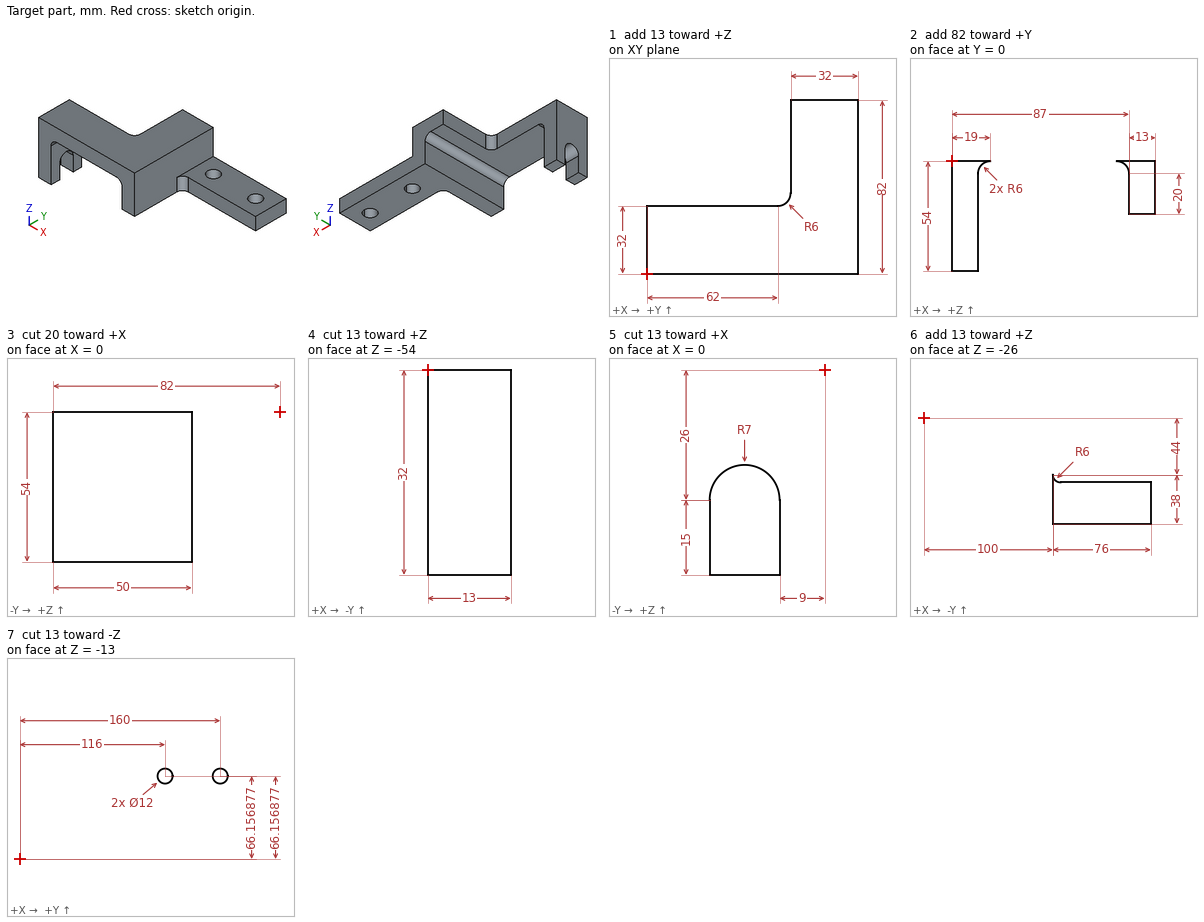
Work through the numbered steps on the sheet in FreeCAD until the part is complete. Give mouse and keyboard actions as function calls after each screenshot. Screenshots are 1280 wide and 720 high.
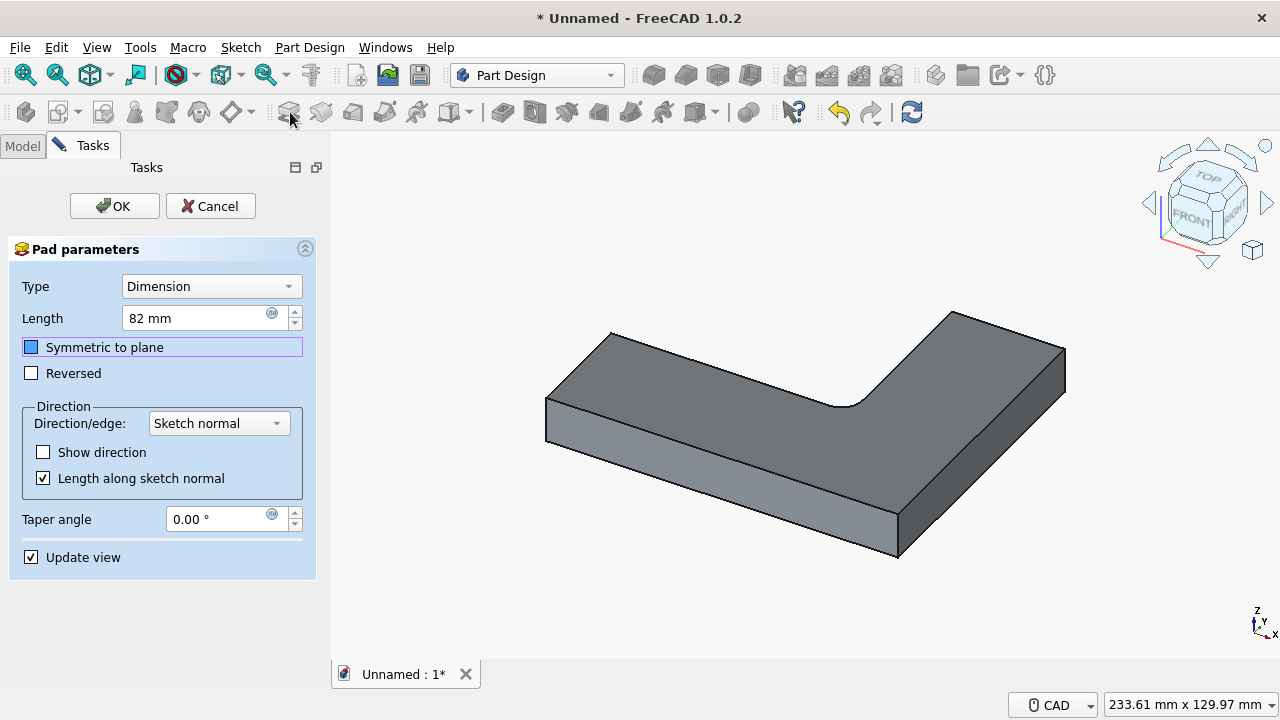
click(30, 373)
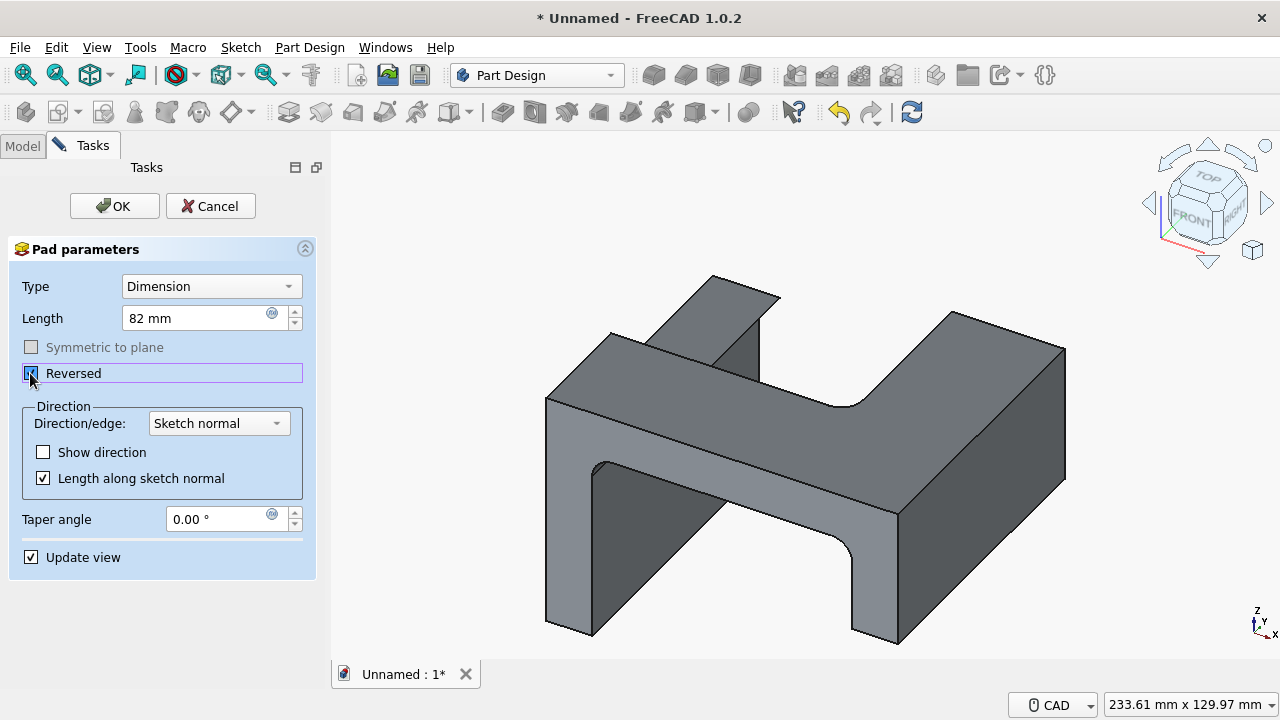
click(115, 206)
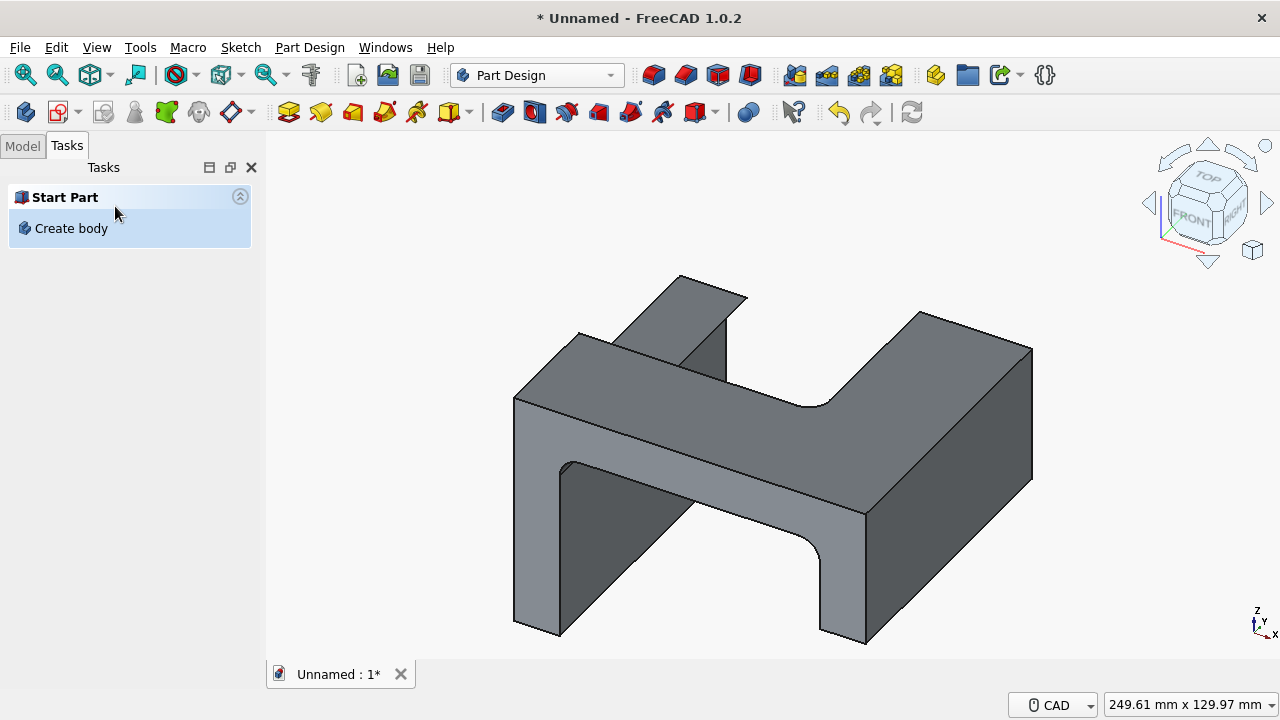
click(26, 76)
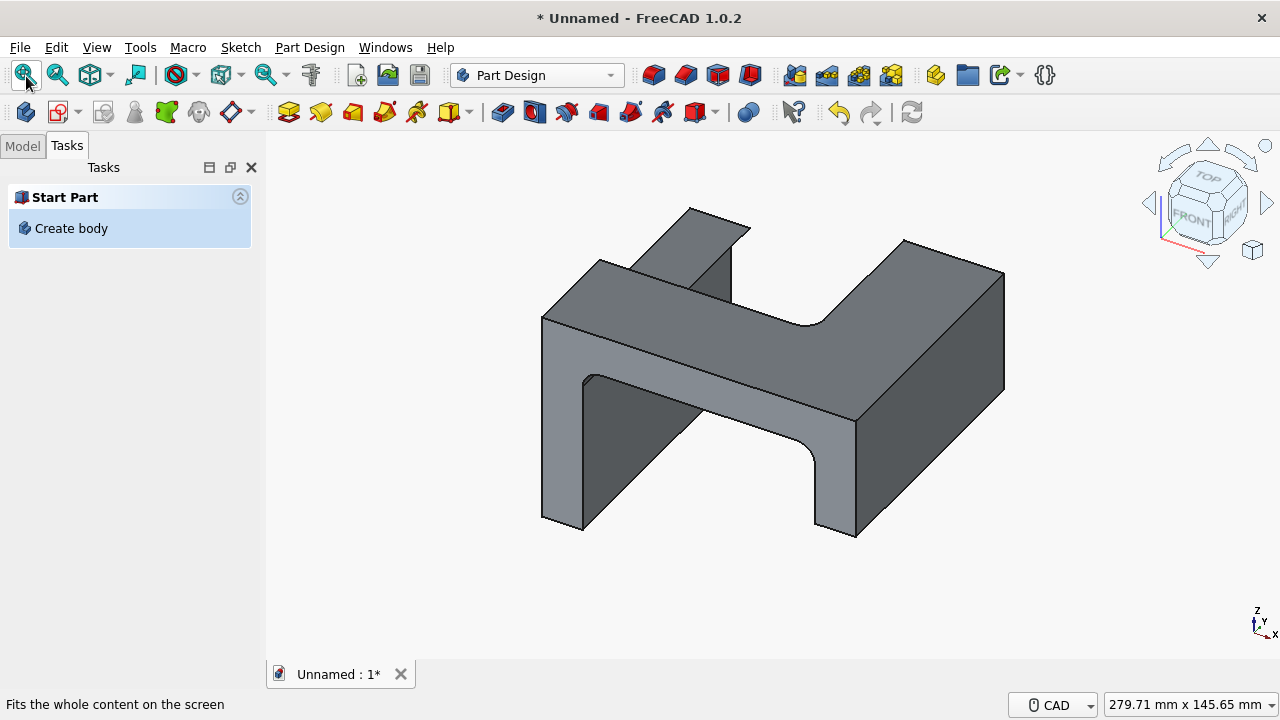
key(6)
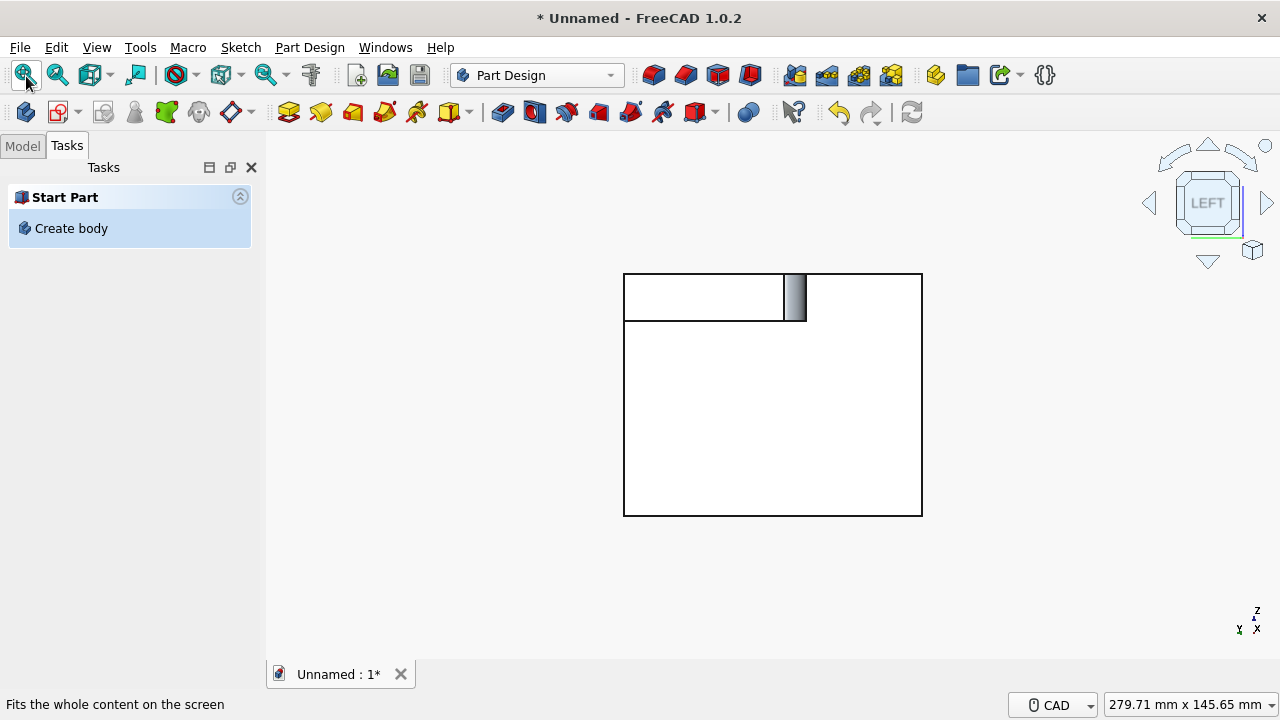
click(731, 429)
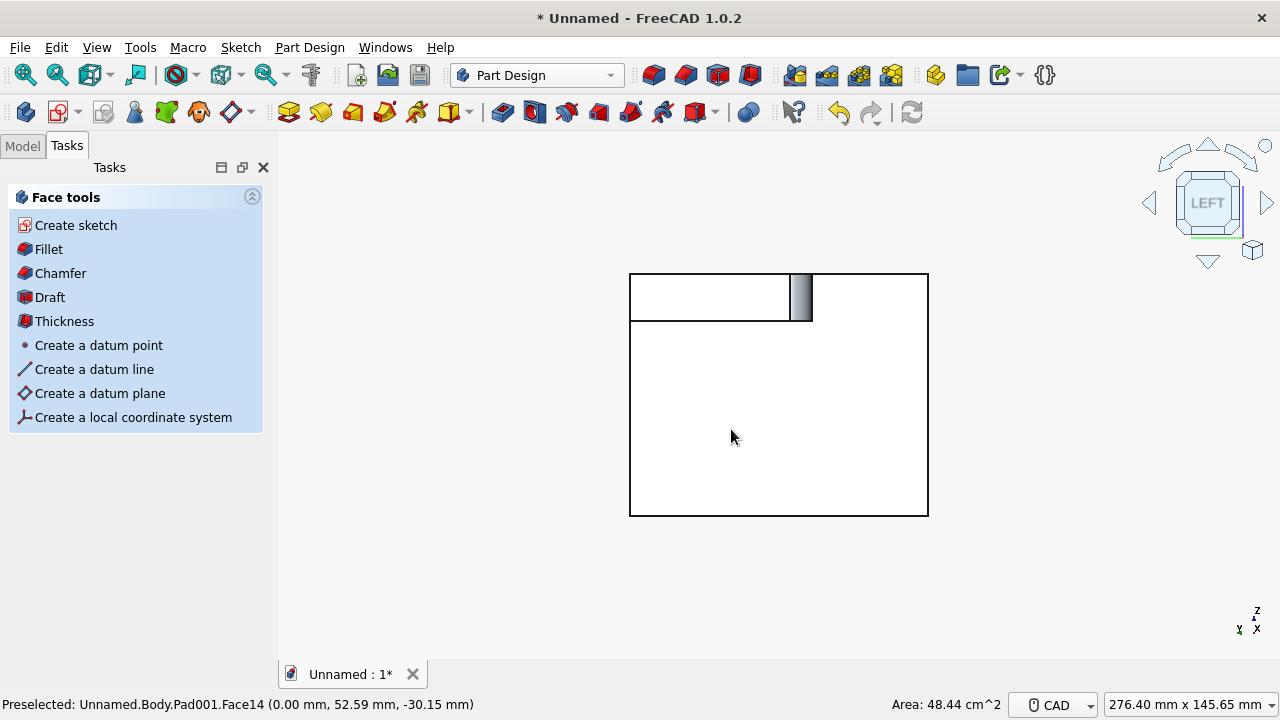
click(58, 112)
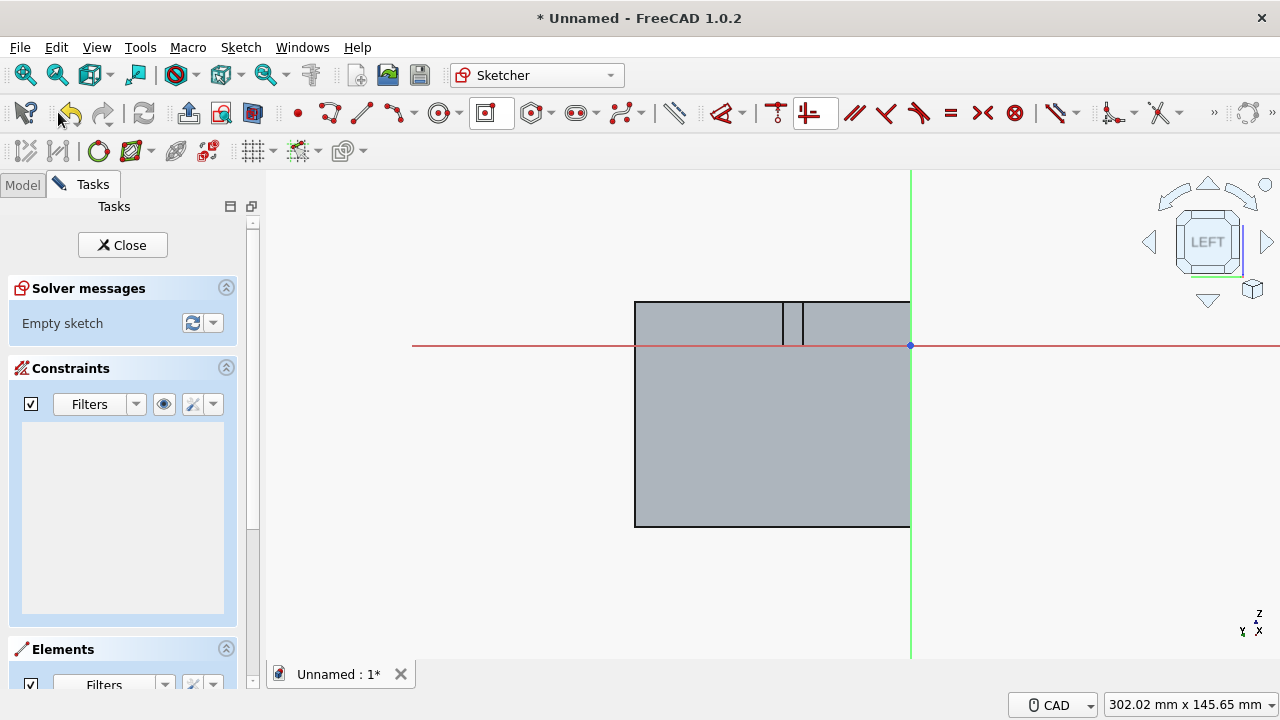
scroll(856, 463, up, 3)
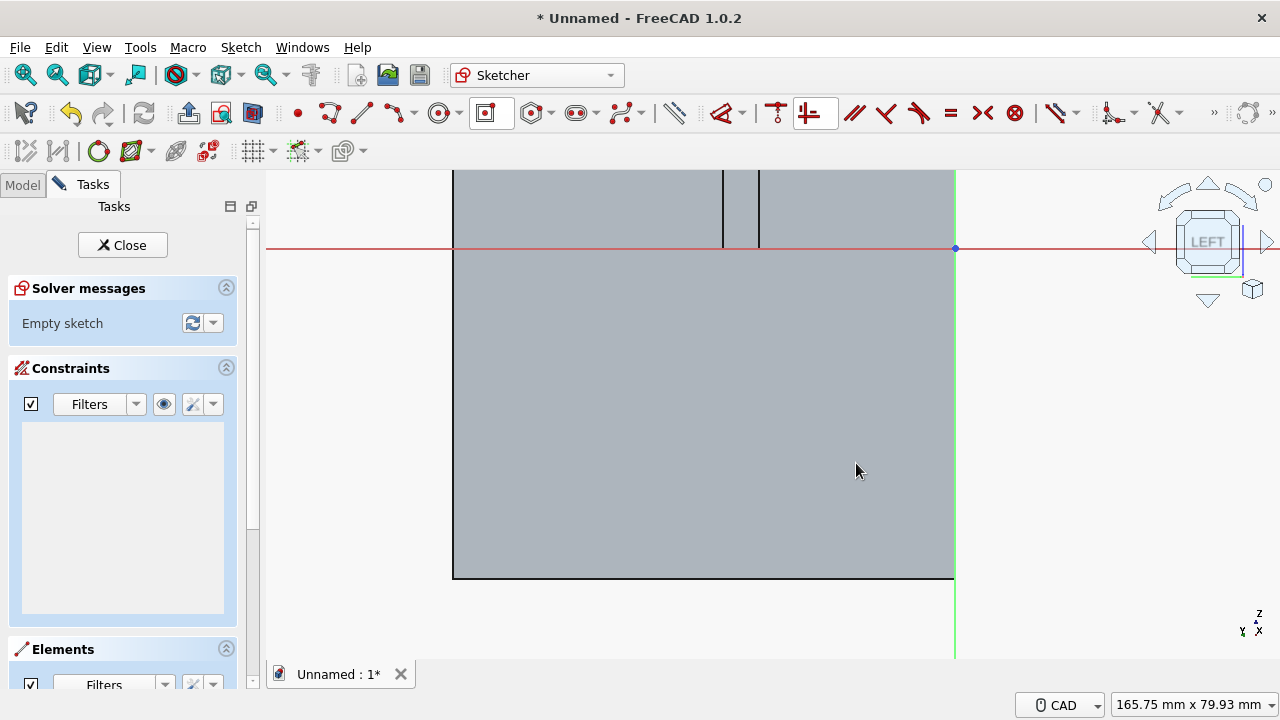
click(508, 114)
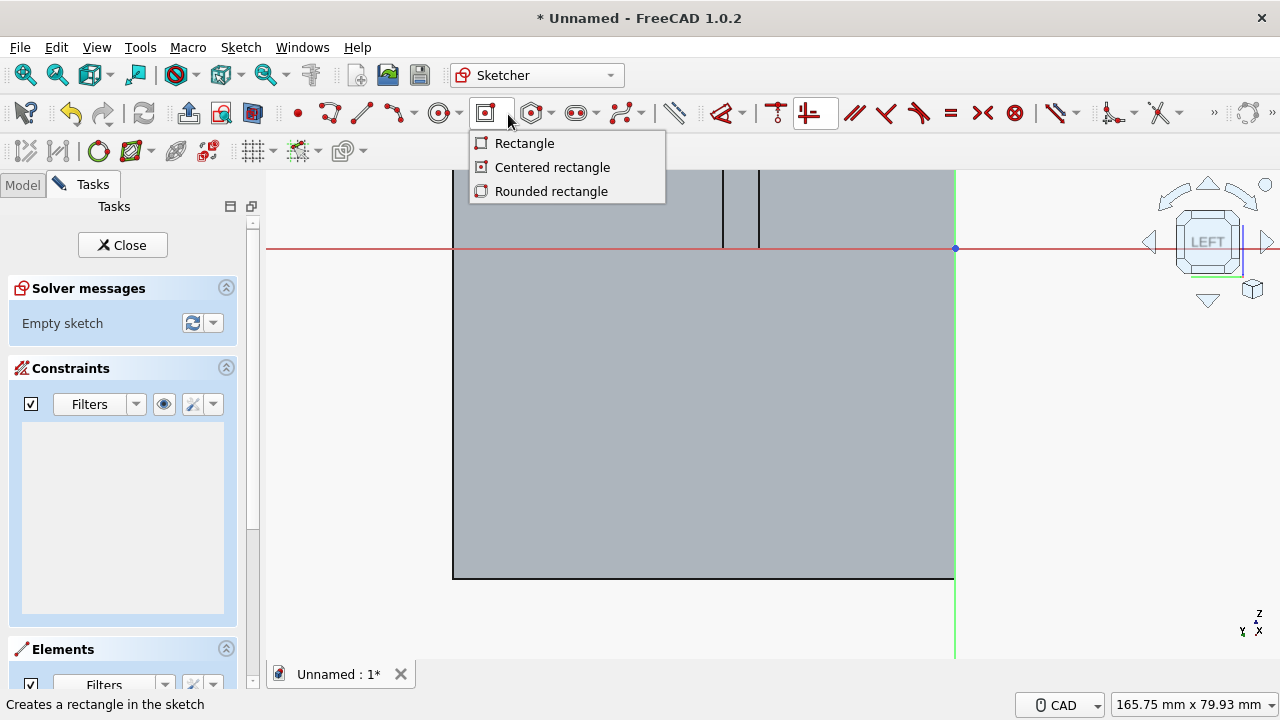
click(568, 143)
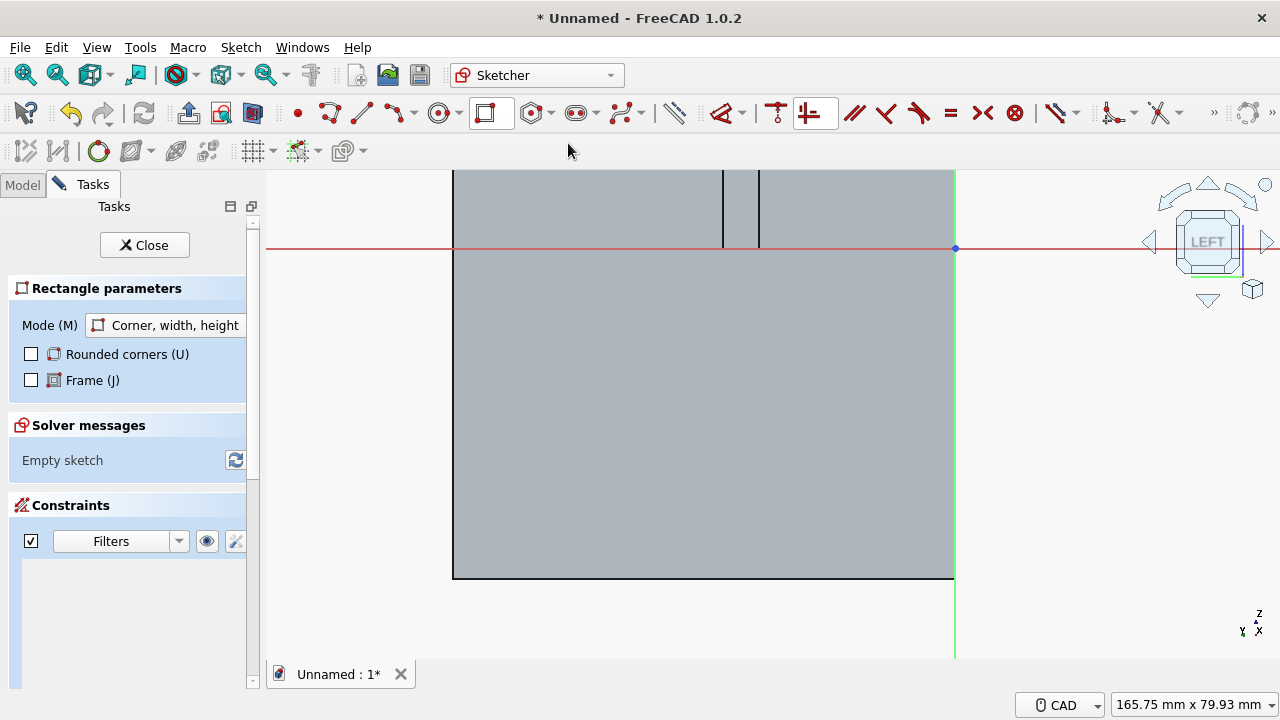
click(453, 249)
click(759, 579)
key(Escape)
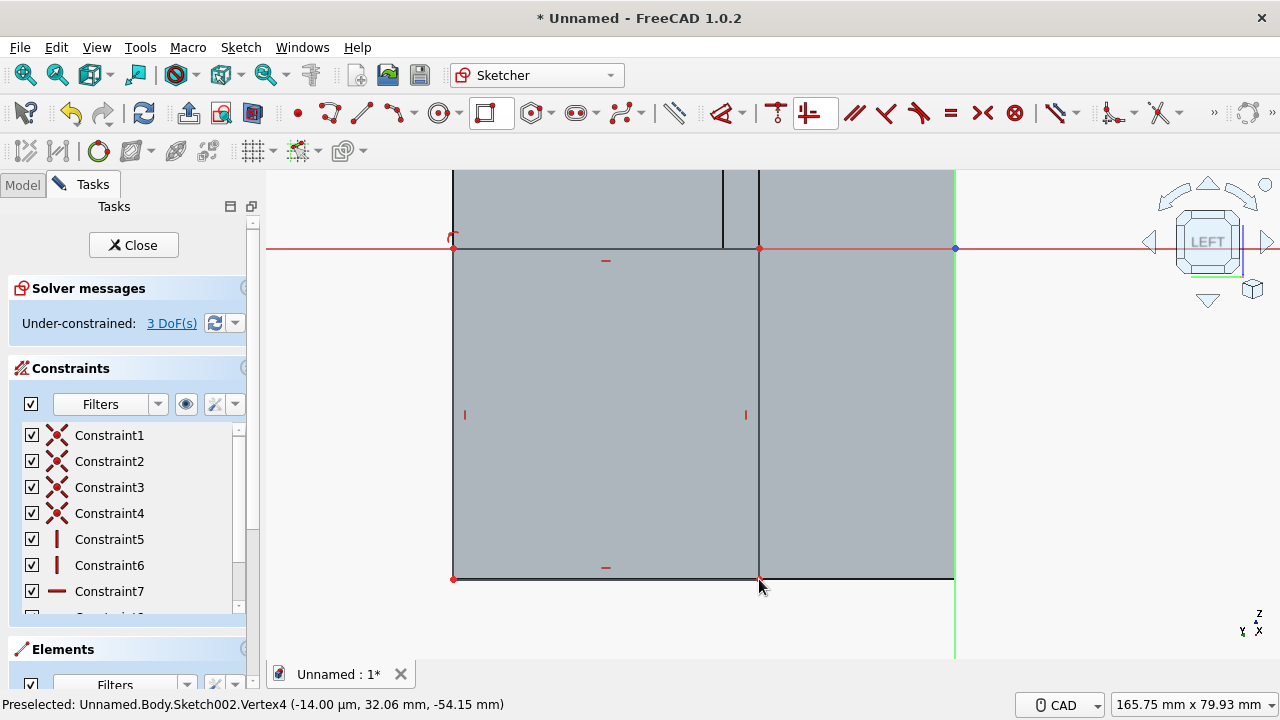
click(722, 114)